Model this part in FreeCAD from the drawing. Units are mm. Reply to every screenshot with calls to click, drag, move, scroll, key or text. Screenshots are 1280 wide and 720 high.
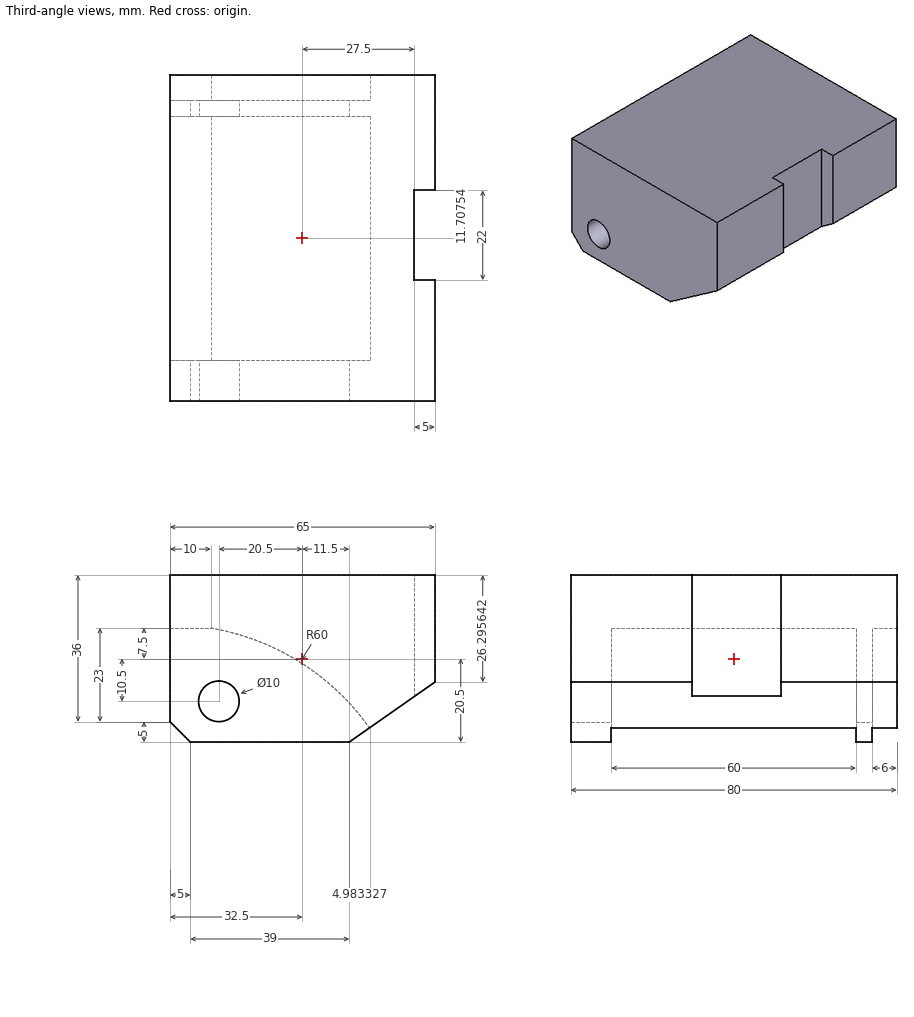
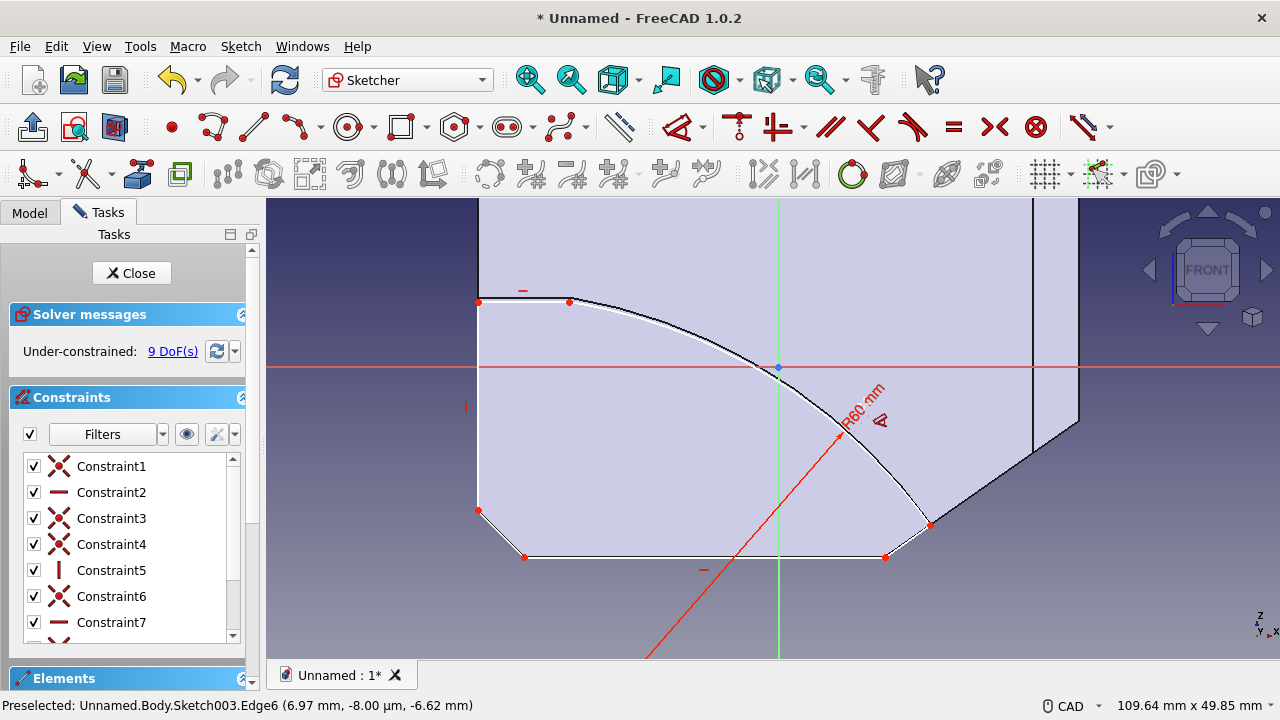
click(777, 558)
click(705, 592)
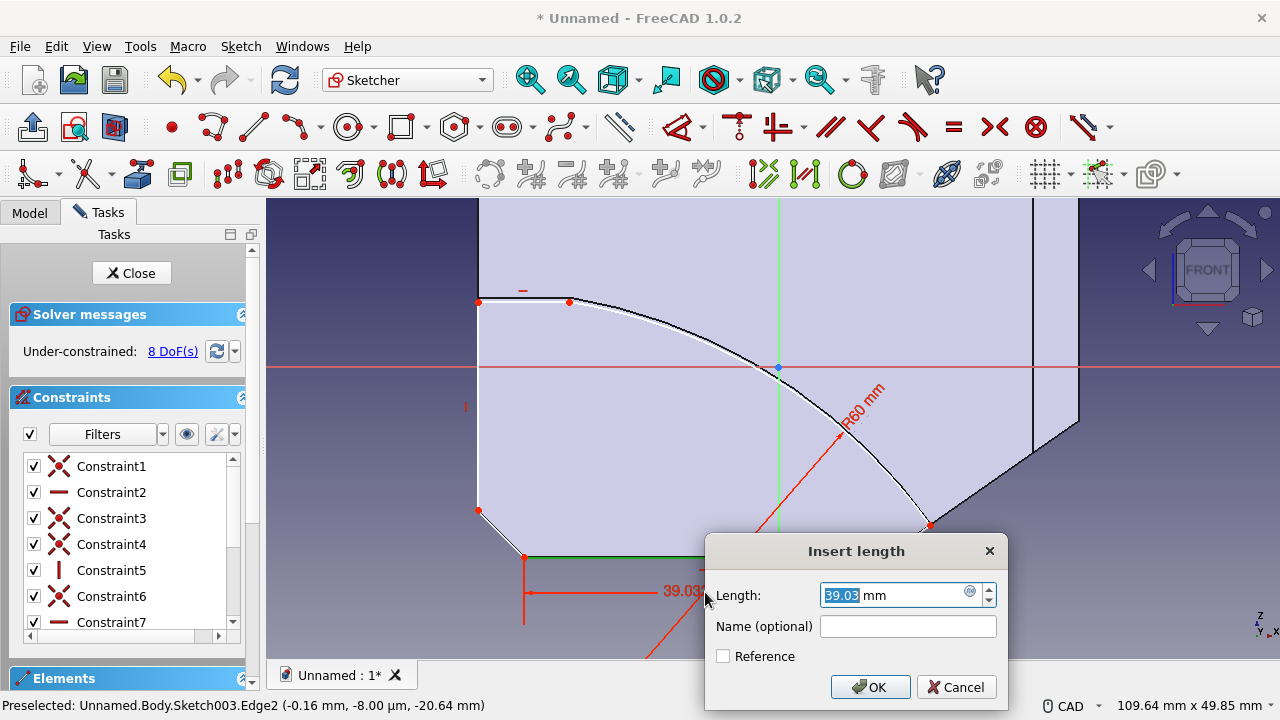
text(39)
key(Return)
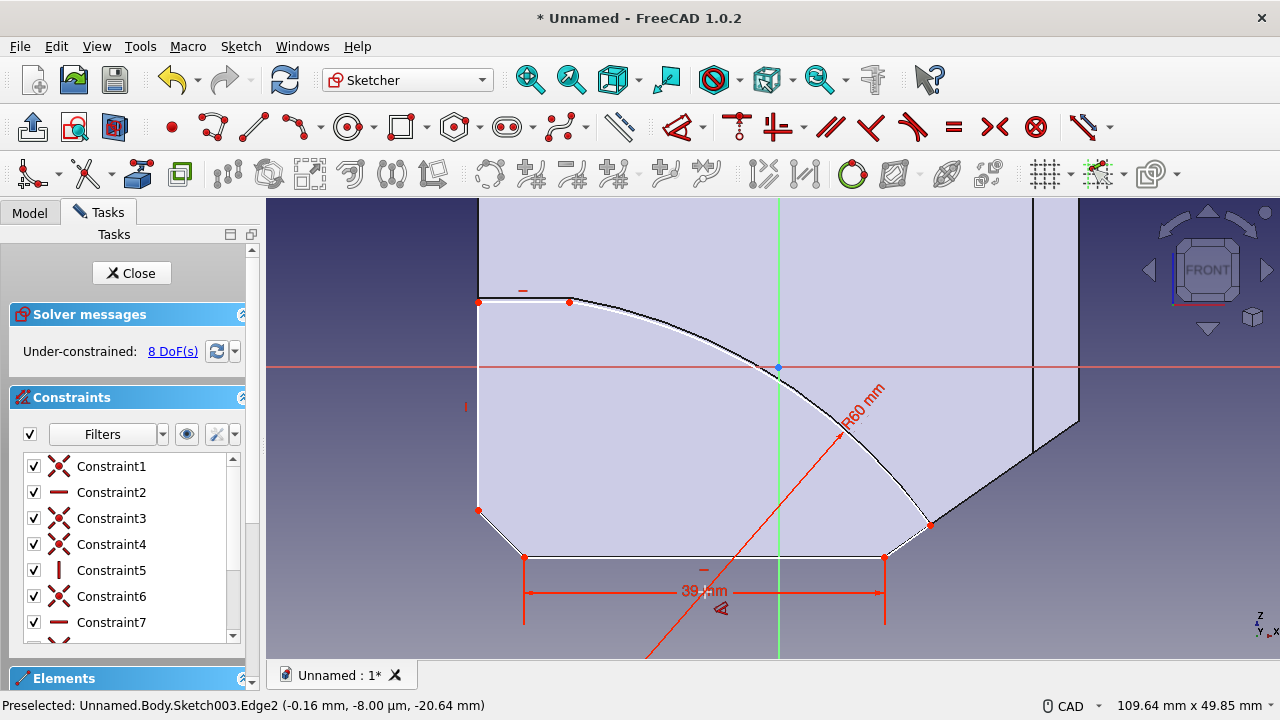
click(478, 448)
click(444, 407)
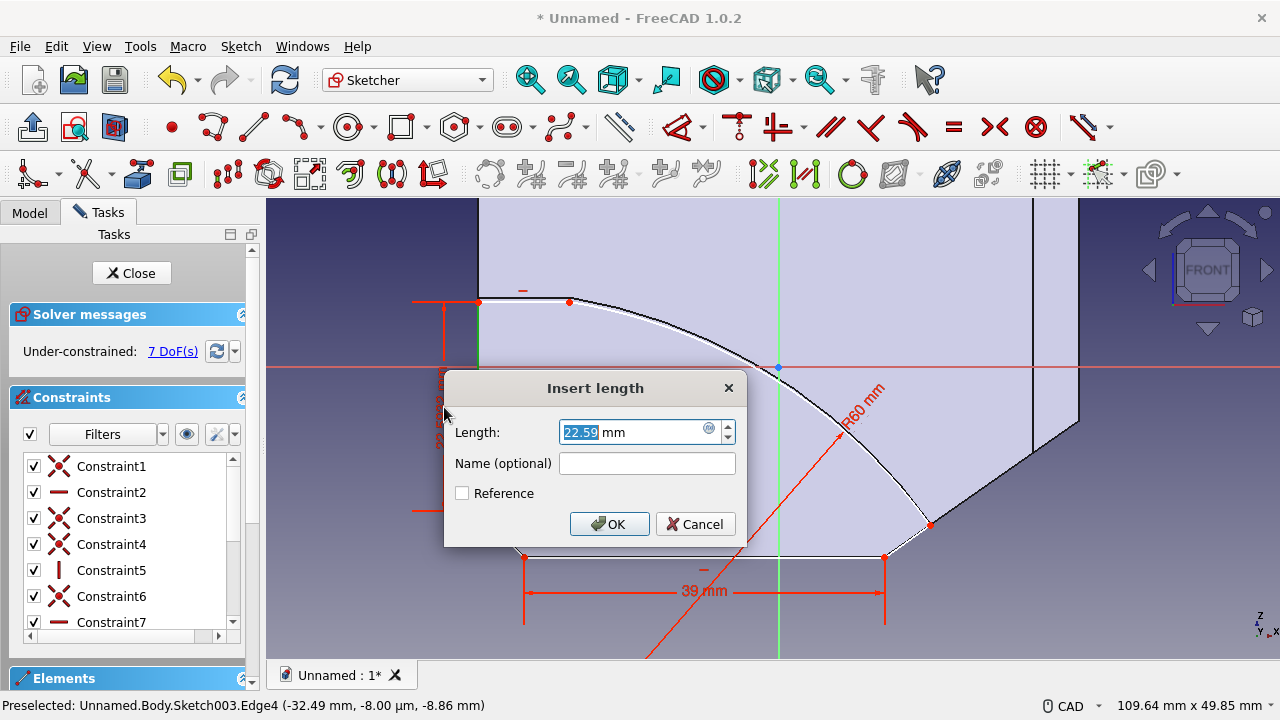
text(23)
key(Return)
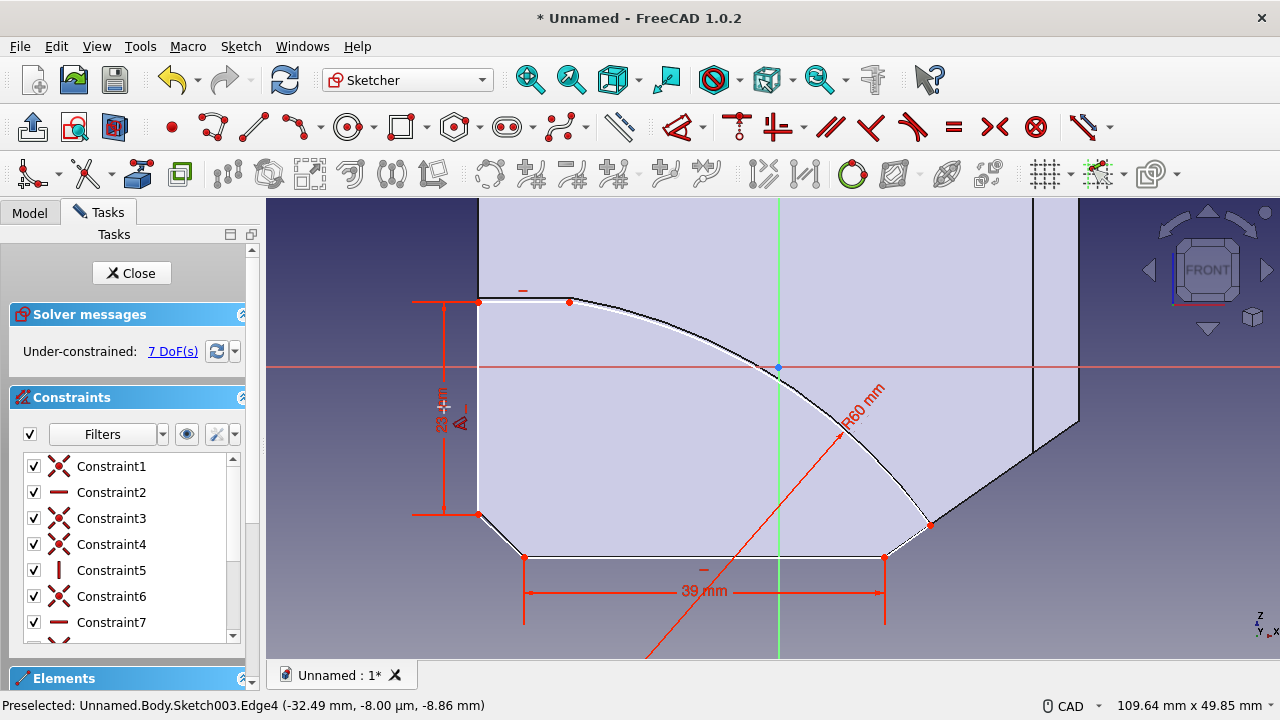
click(506, 302)
click(524, 268)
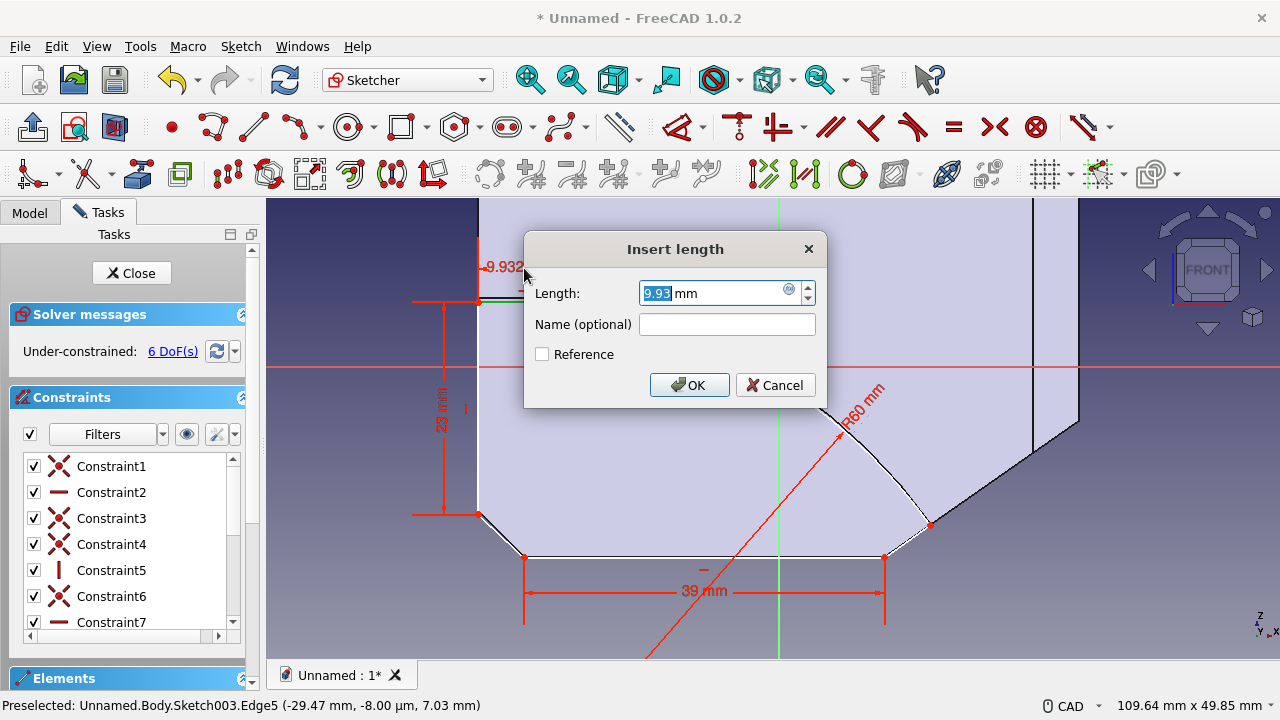
text(10)
key(Return)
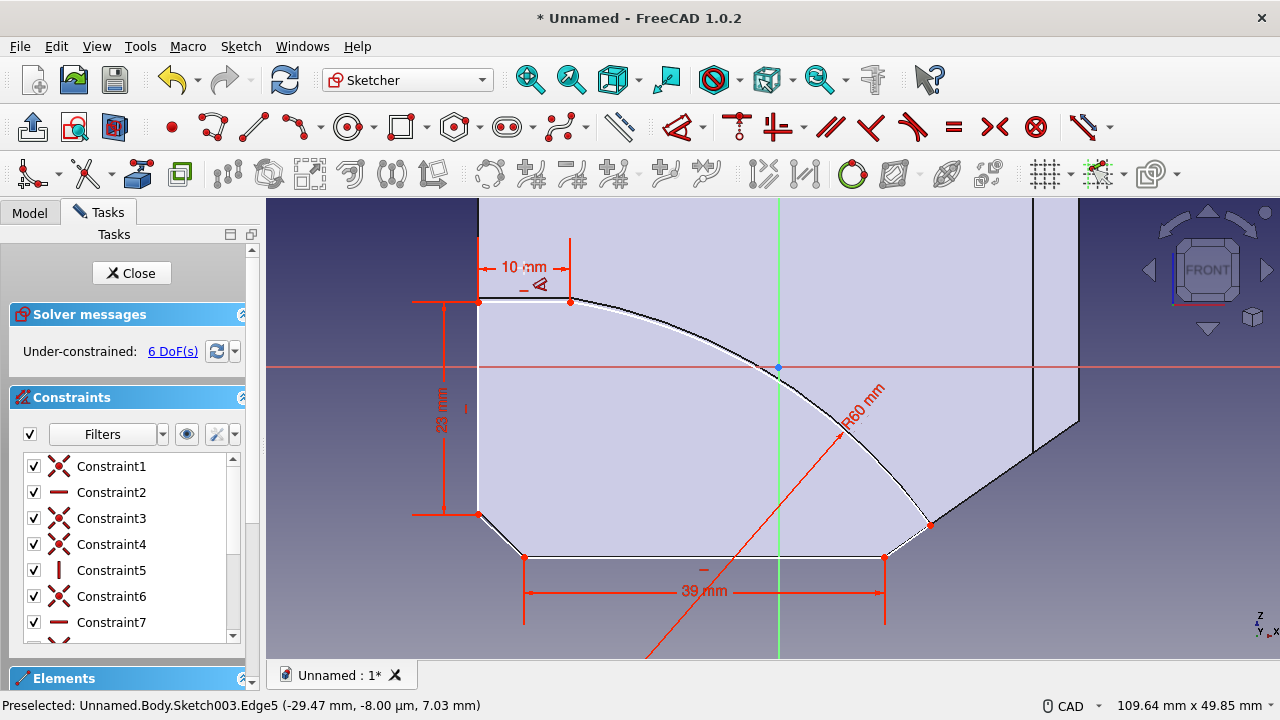
click(510, 545)
click(501, 592)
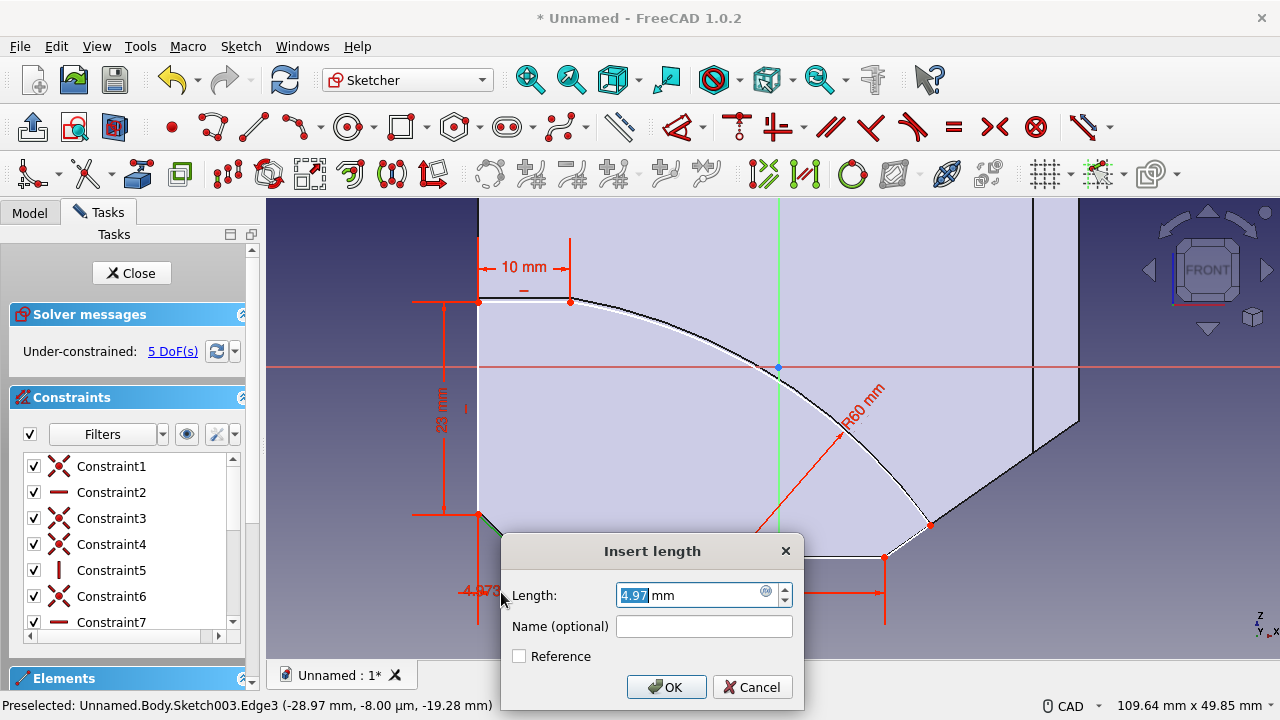
text(5)
key(Return)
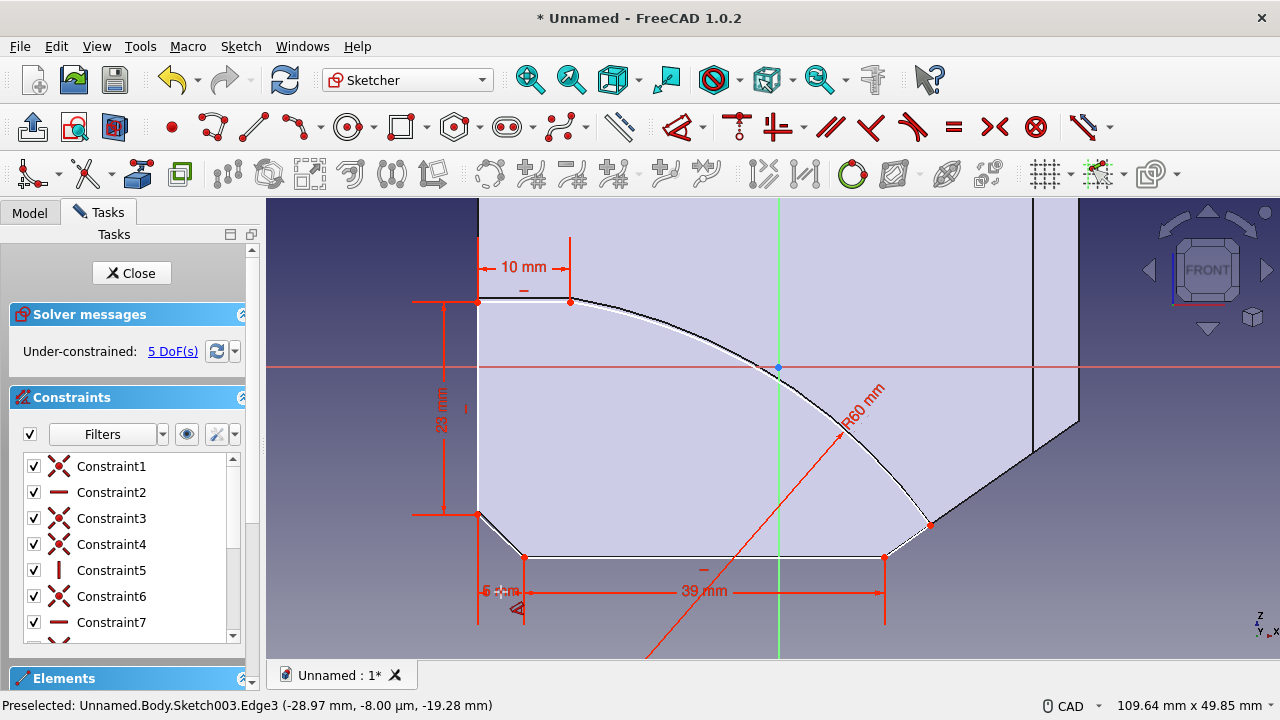
click(510, 545)
click(444, 536)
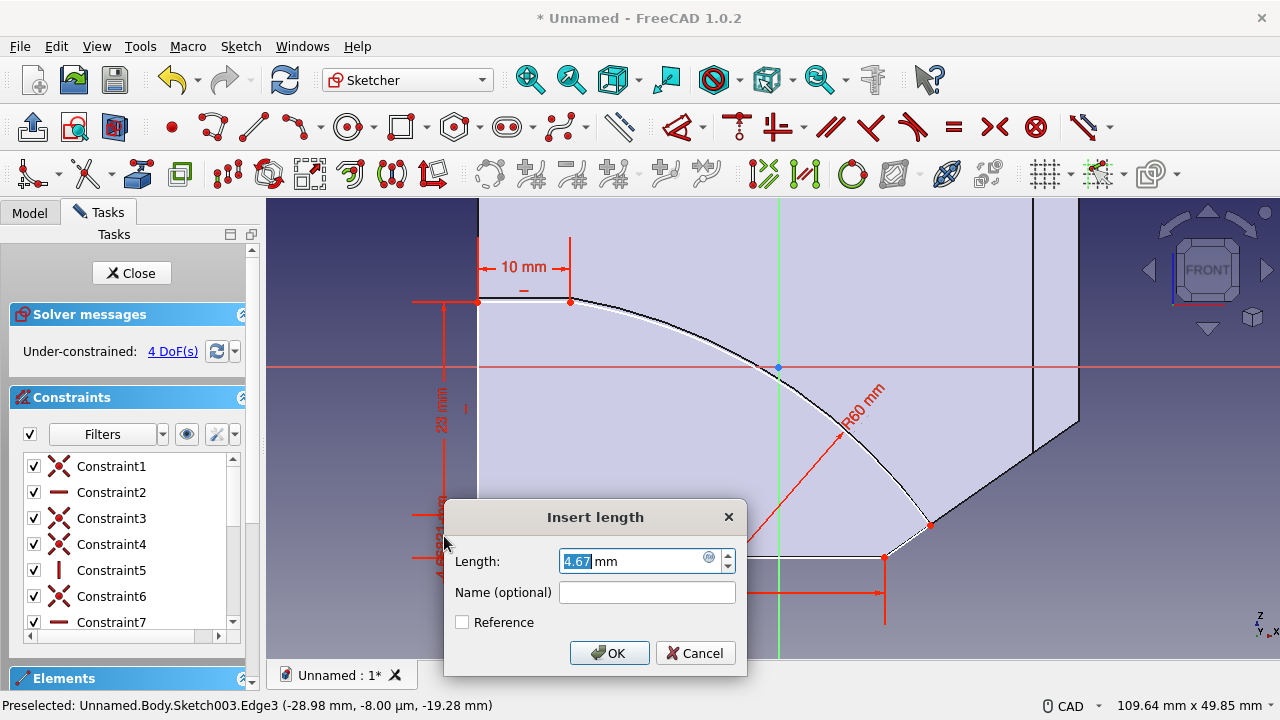
text(5)
key(Return)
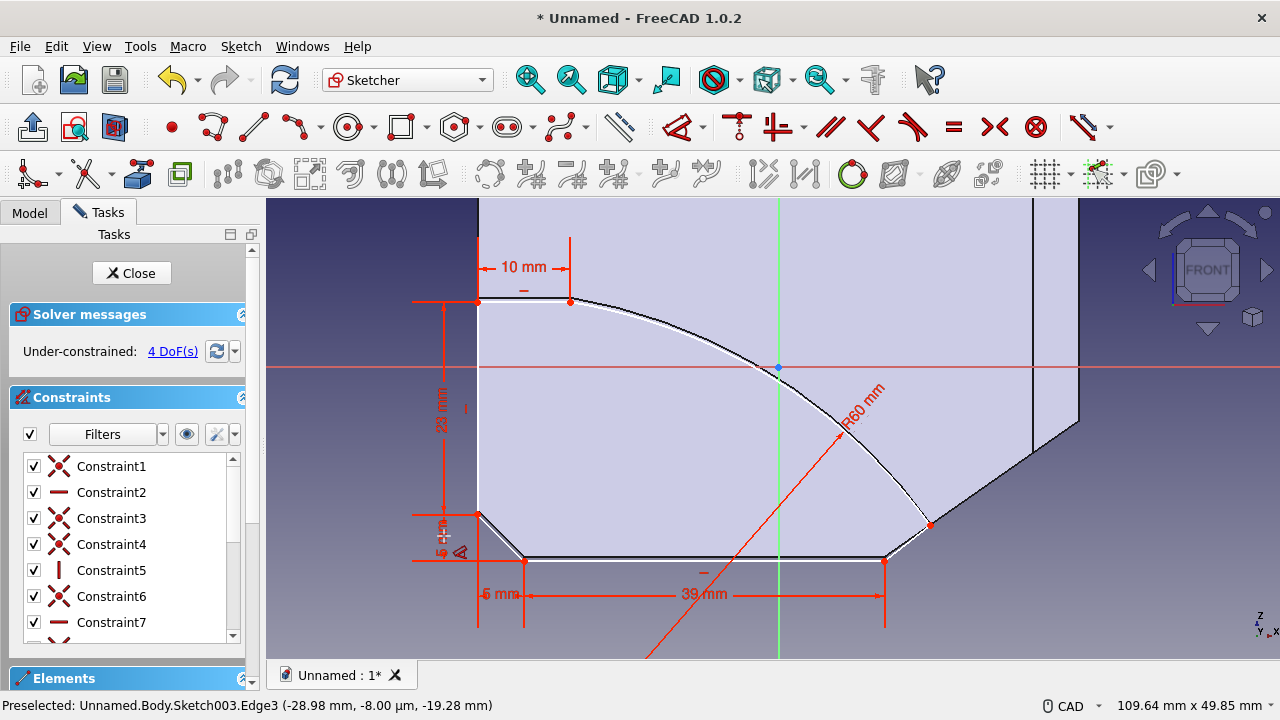
click(478, 302)
click(444, 335)